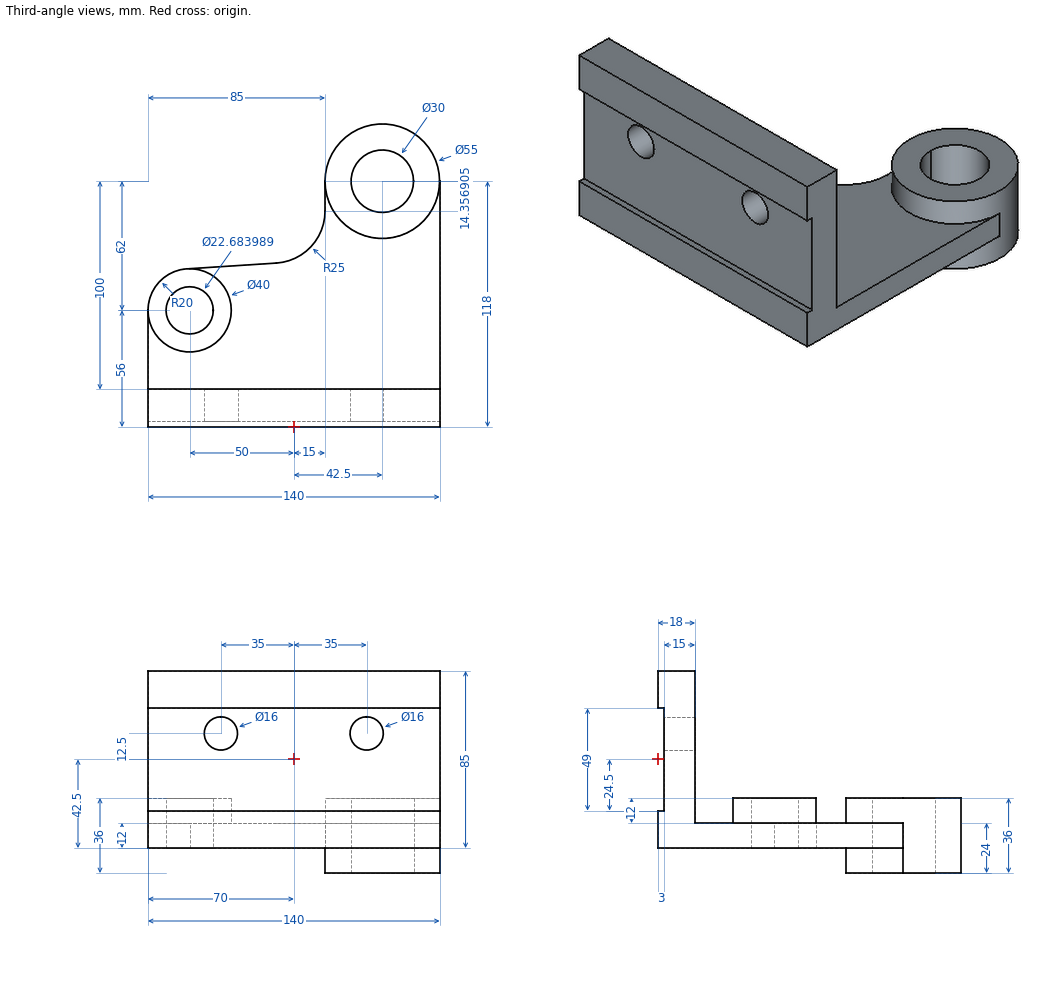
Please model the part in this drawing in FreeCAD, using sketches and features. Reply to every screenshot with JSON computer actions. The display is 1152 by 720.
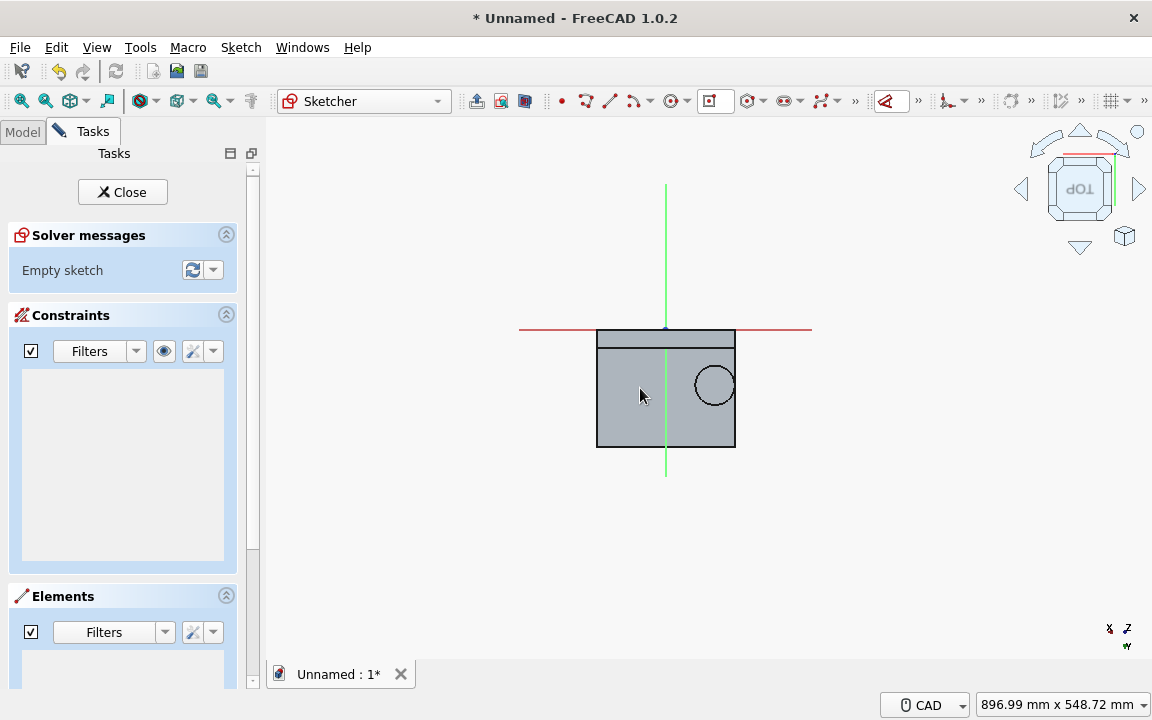
{"action": "scroll", "coordinate": [620, 458], "scroll_direction": "up", "scroll_amount": 9}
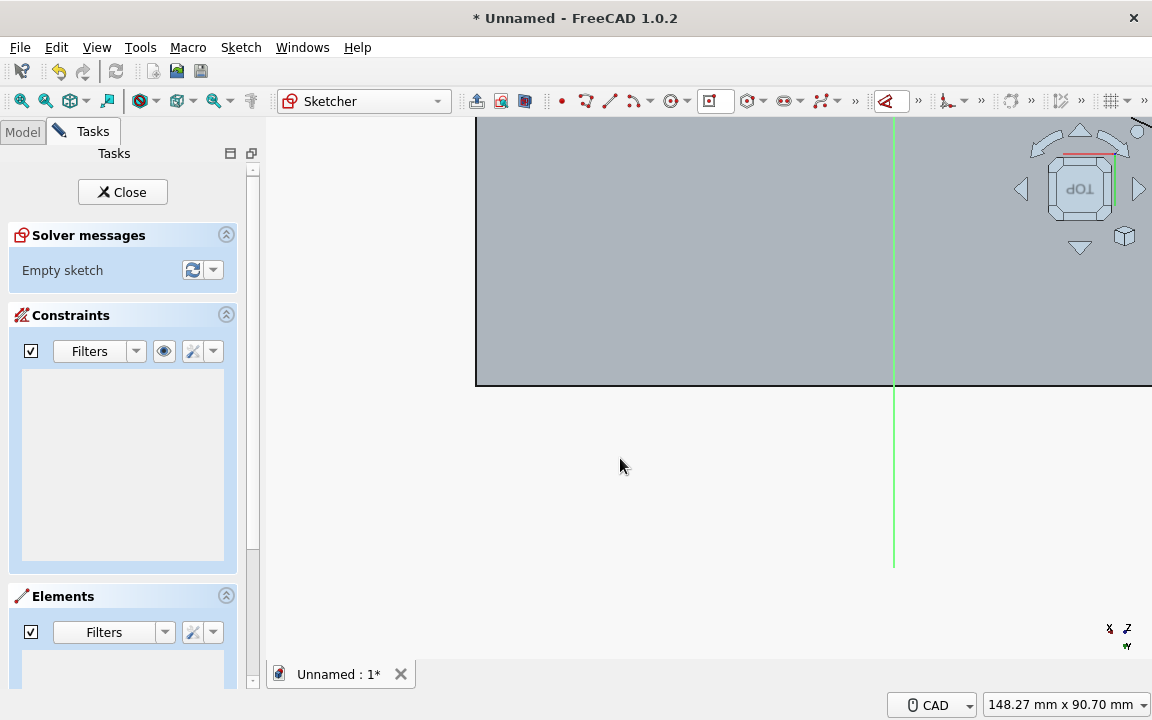
{"action": "key", "text": "g c"}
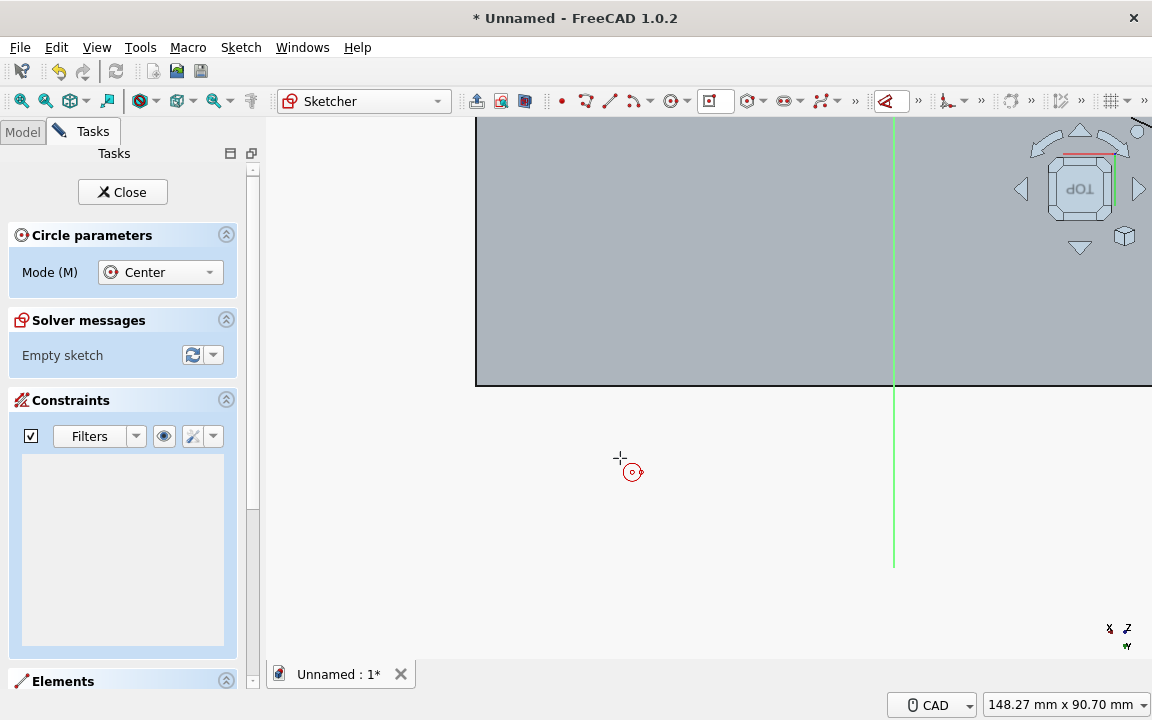
{"action": "left_click", "coordinate": [640, 386]}
{"action": "left_click", "coordinate": [756, 270]}
{"action": "key", "text": "Escape"}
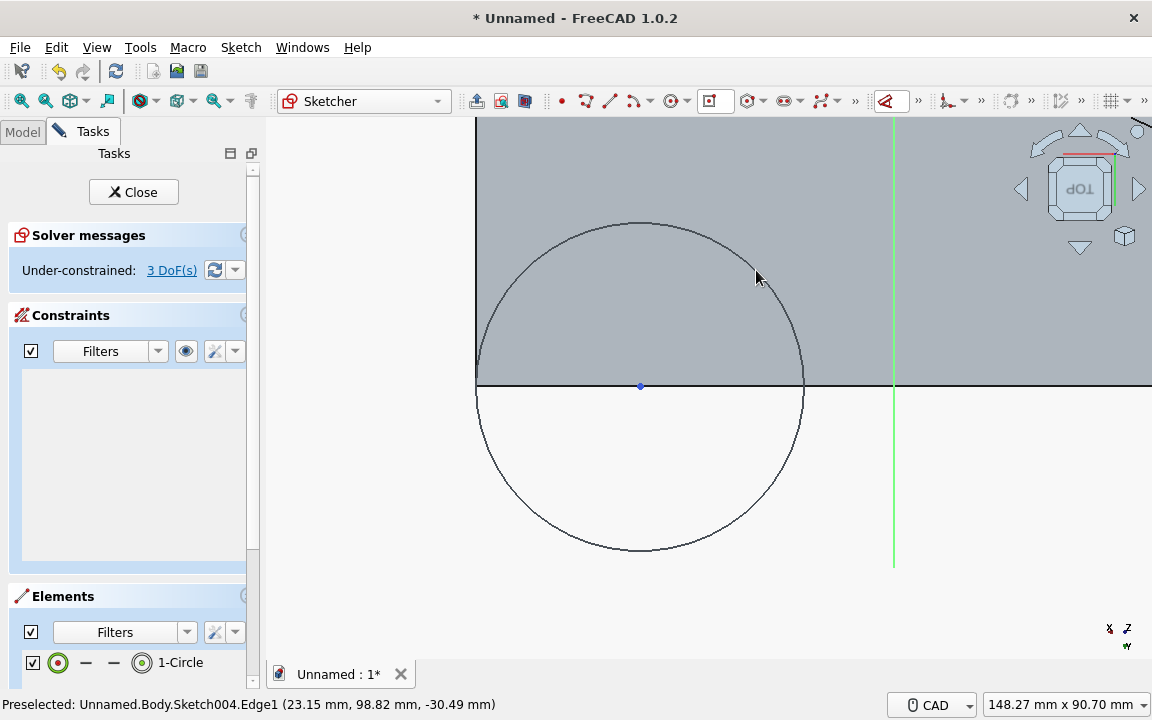
{"action": "left_click", "coordinate": [756, 271]}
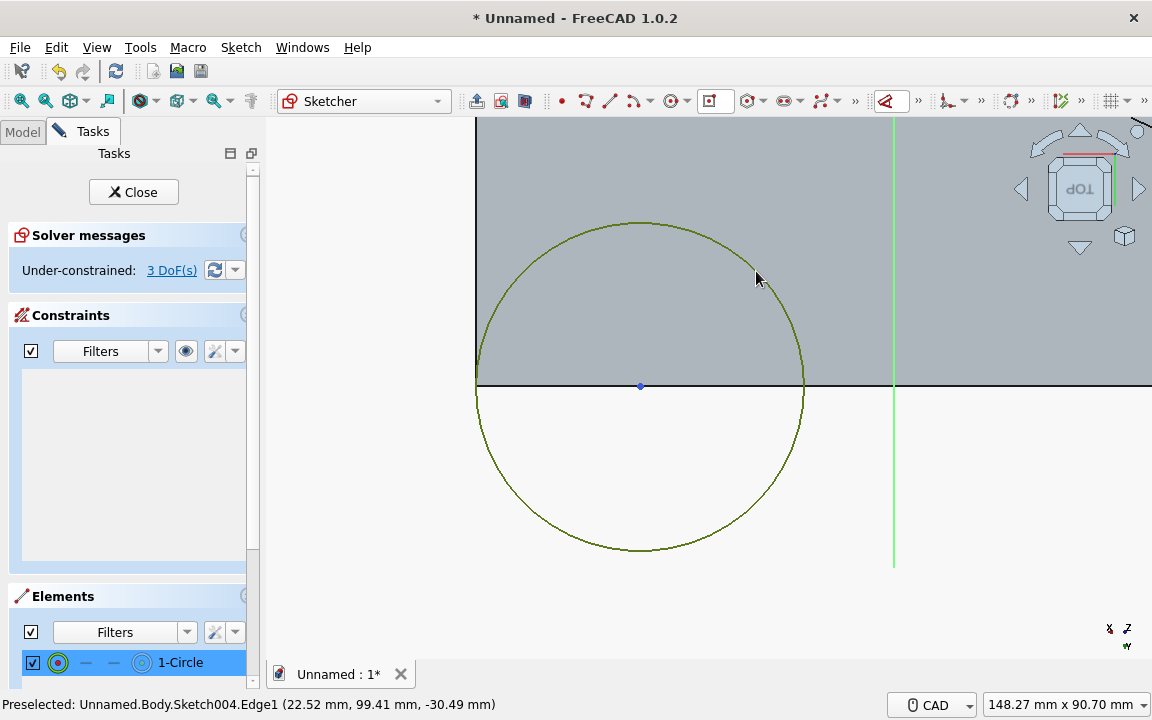
{"action": "key", "text": "k o"}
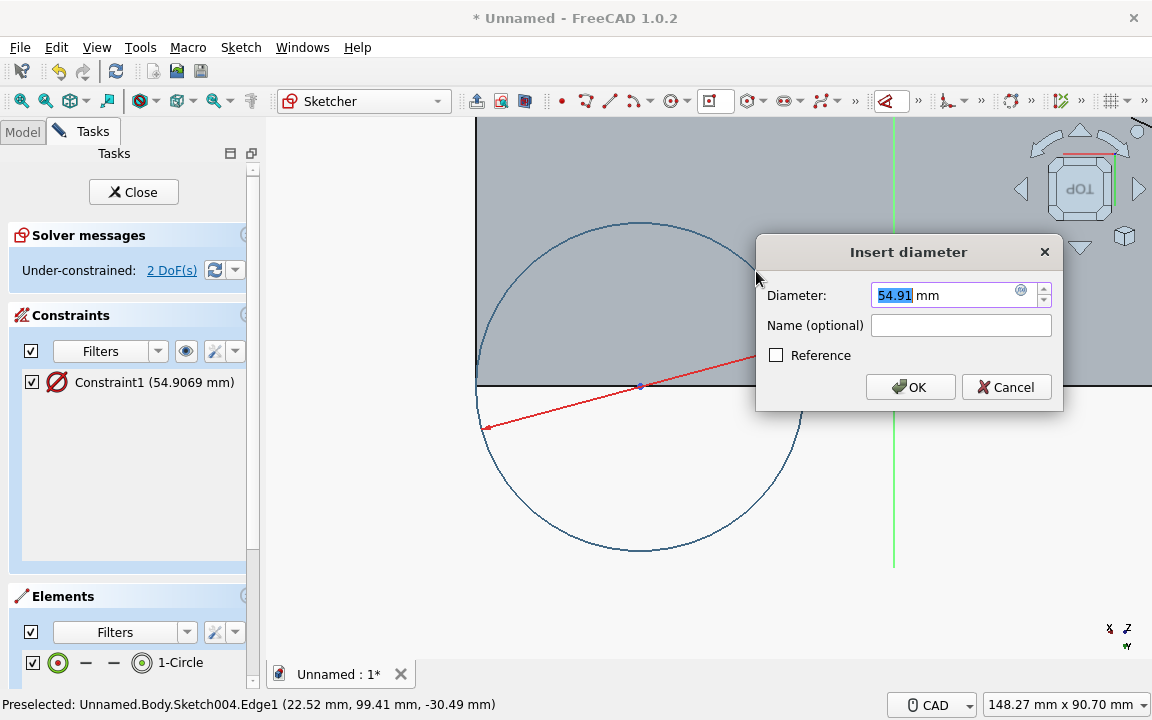
{"action": "type", "text": "55"}
{"action": "key", "text": "Return"}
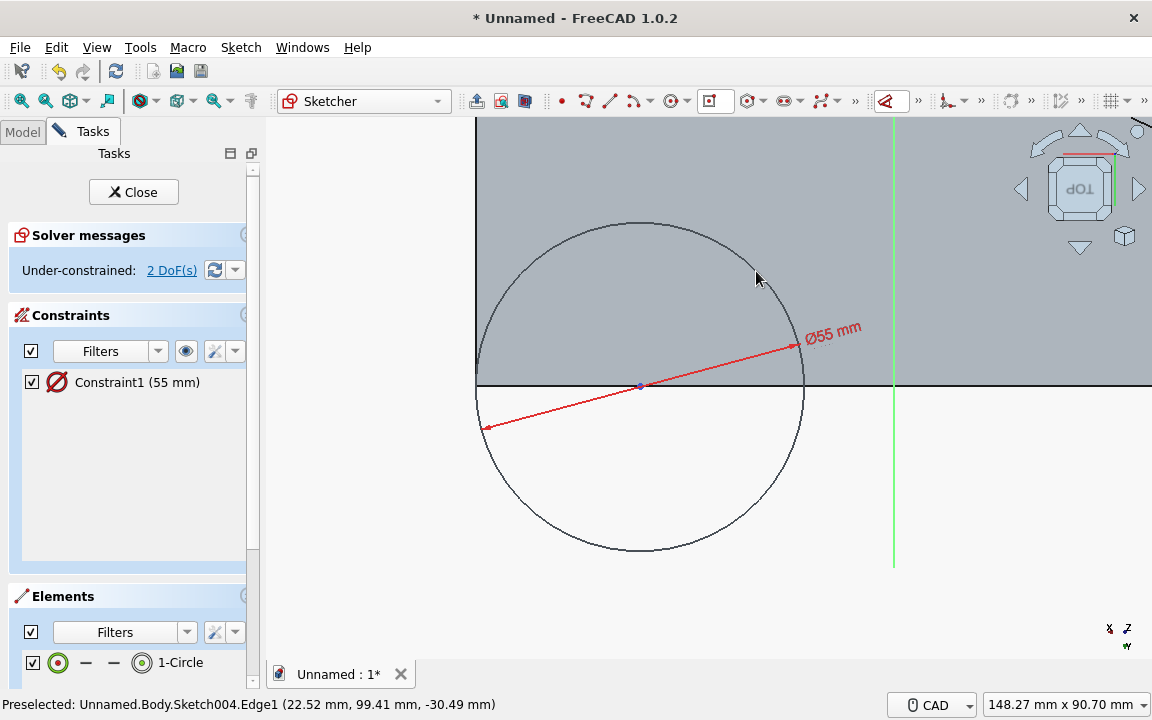
{"action": "left_click", "coordinate": [640, 387]}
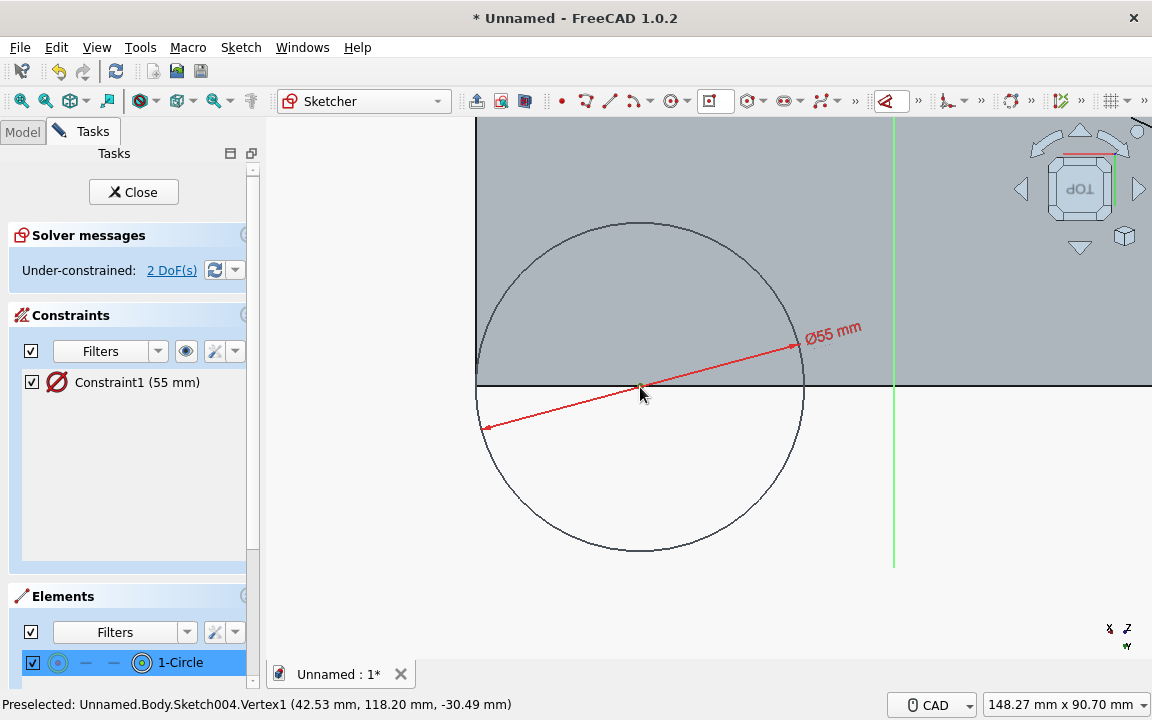
{"action": "key", "text": "i"}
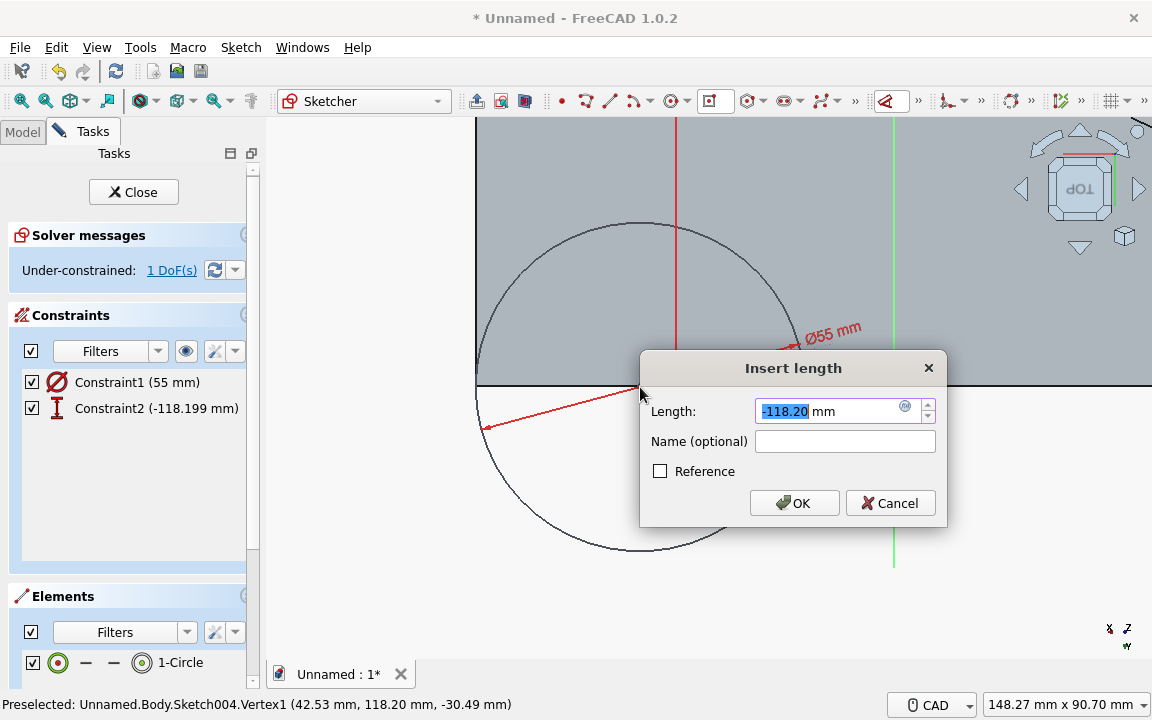
{"action": "type", "text": "-118"}
{"action": "key", "text": "Return"}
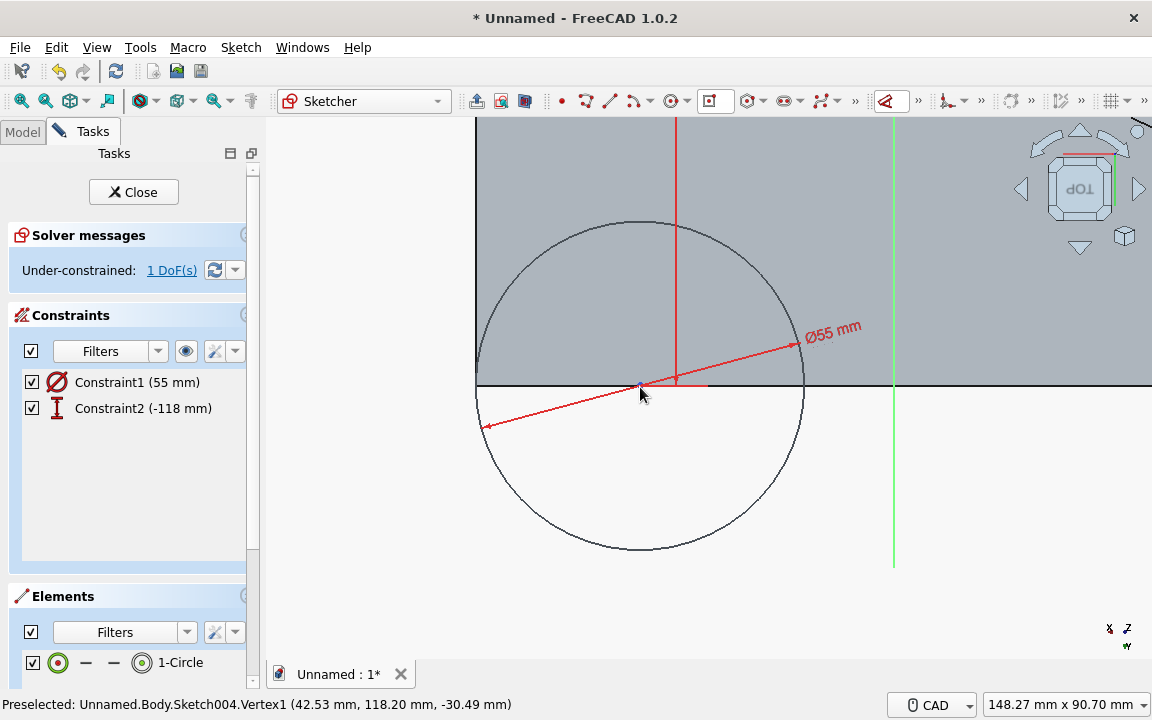
{"action": "left_click", "coordinate": [640, 386]}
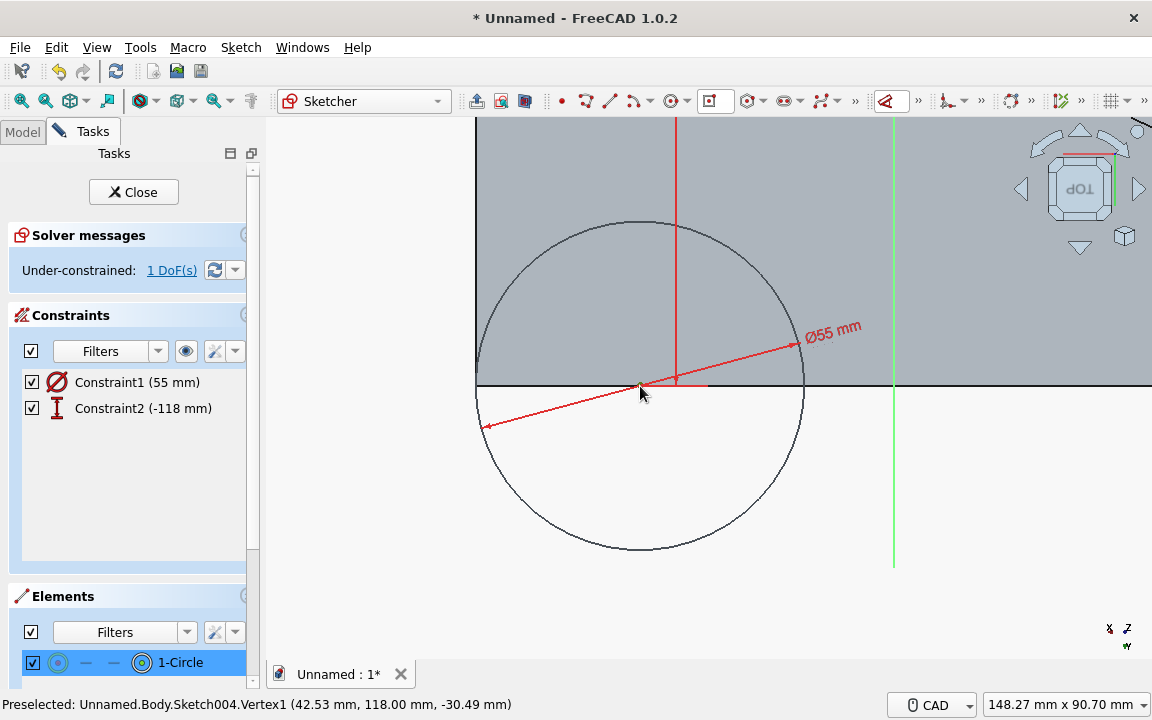
{"action": "key", "text": "l"}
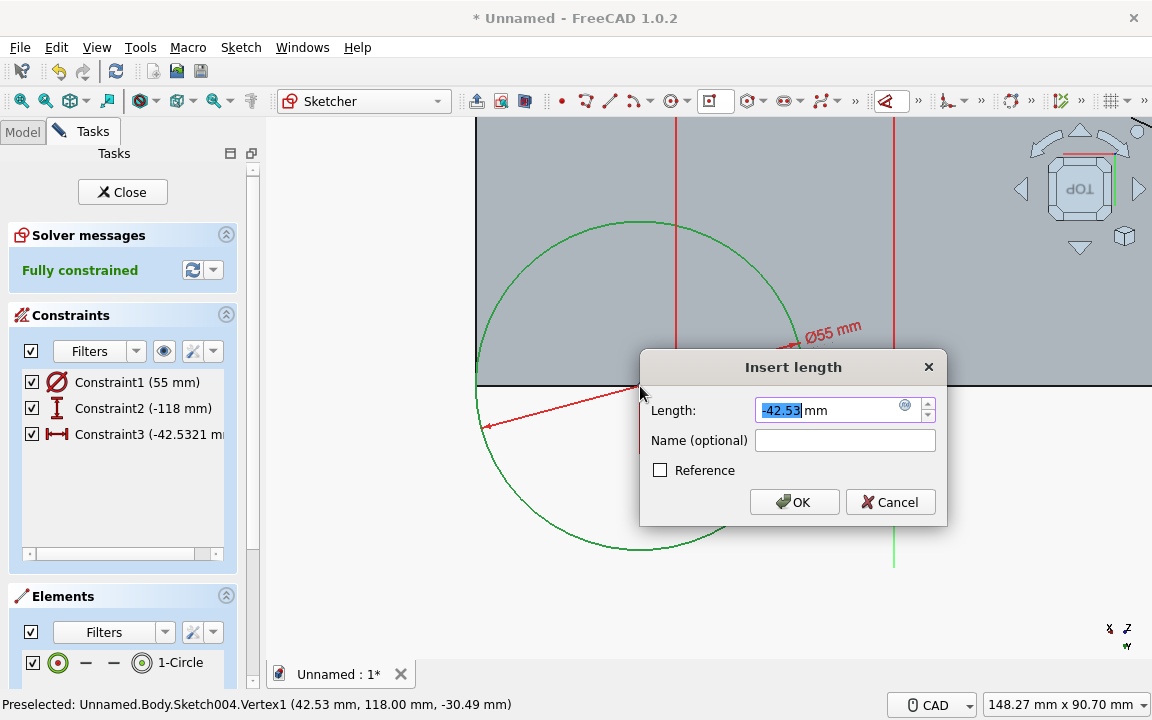
{"action": "type", "text": "-42.5"}
{"action": "key", "text": "Return"}